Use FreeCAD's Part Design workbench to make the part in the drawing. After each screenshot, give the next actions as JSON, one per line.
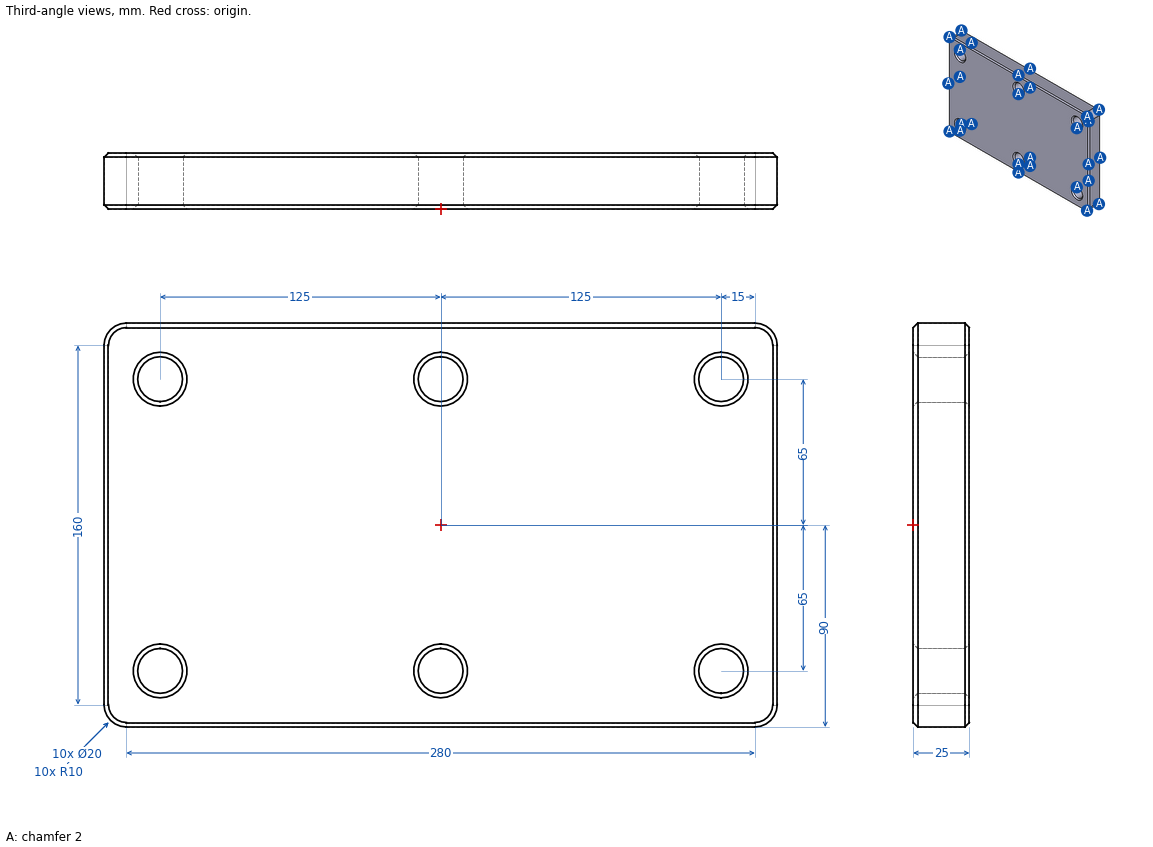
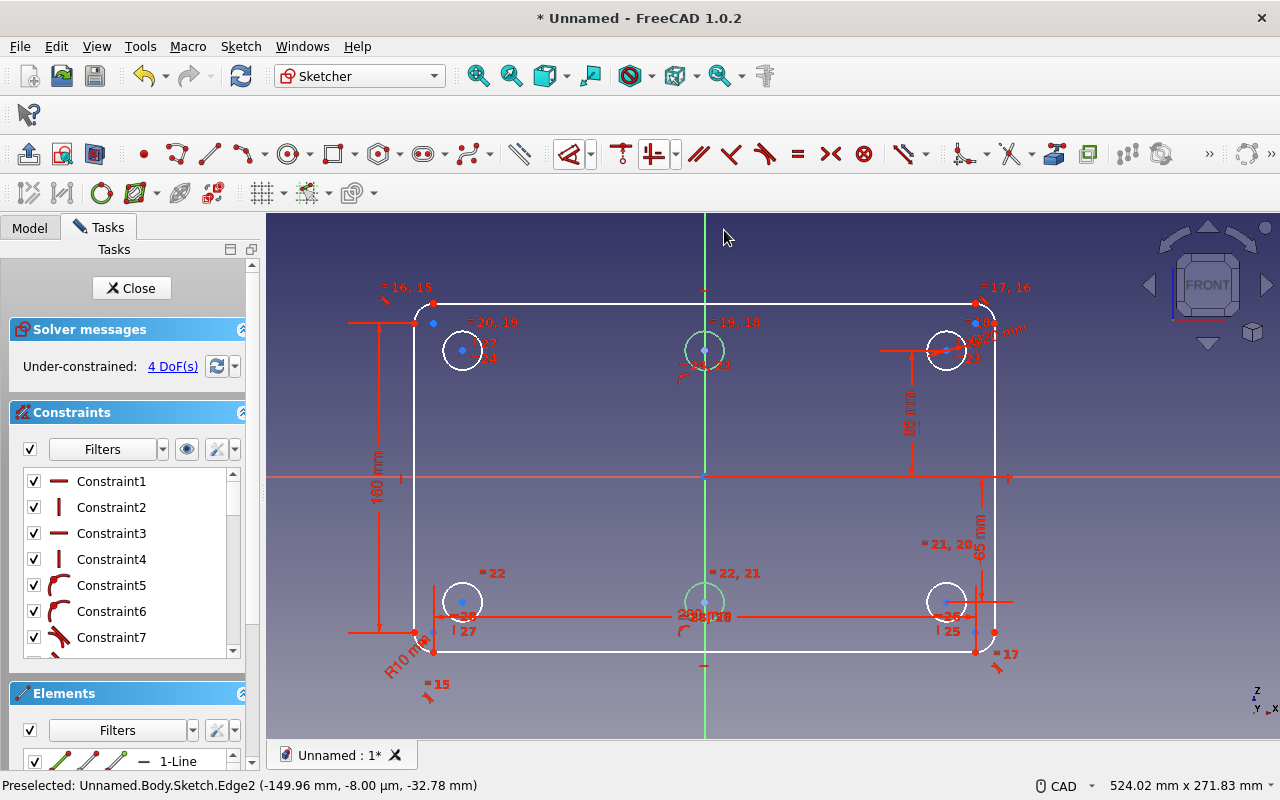
{"action": "left_click", "coordinate": [976, 652]}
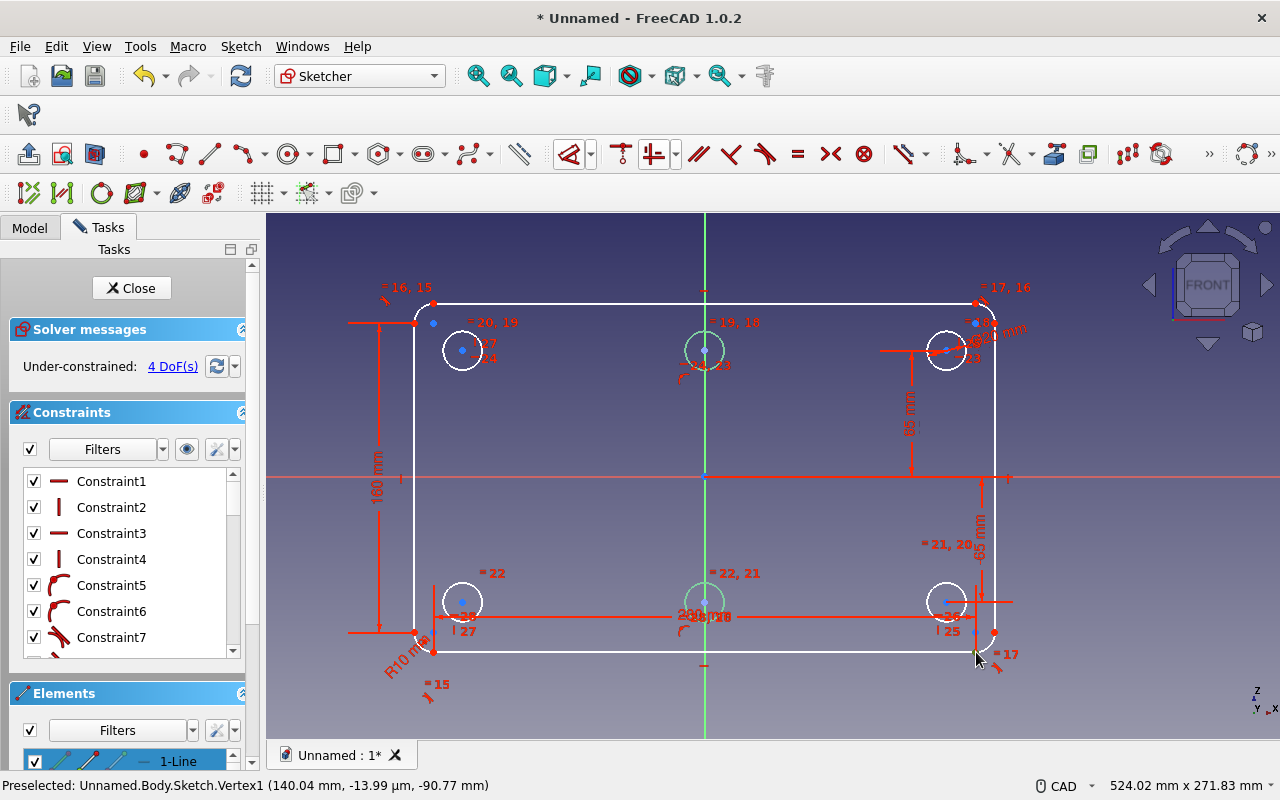
{"action": "left_click", "coordinate": [590, 154]}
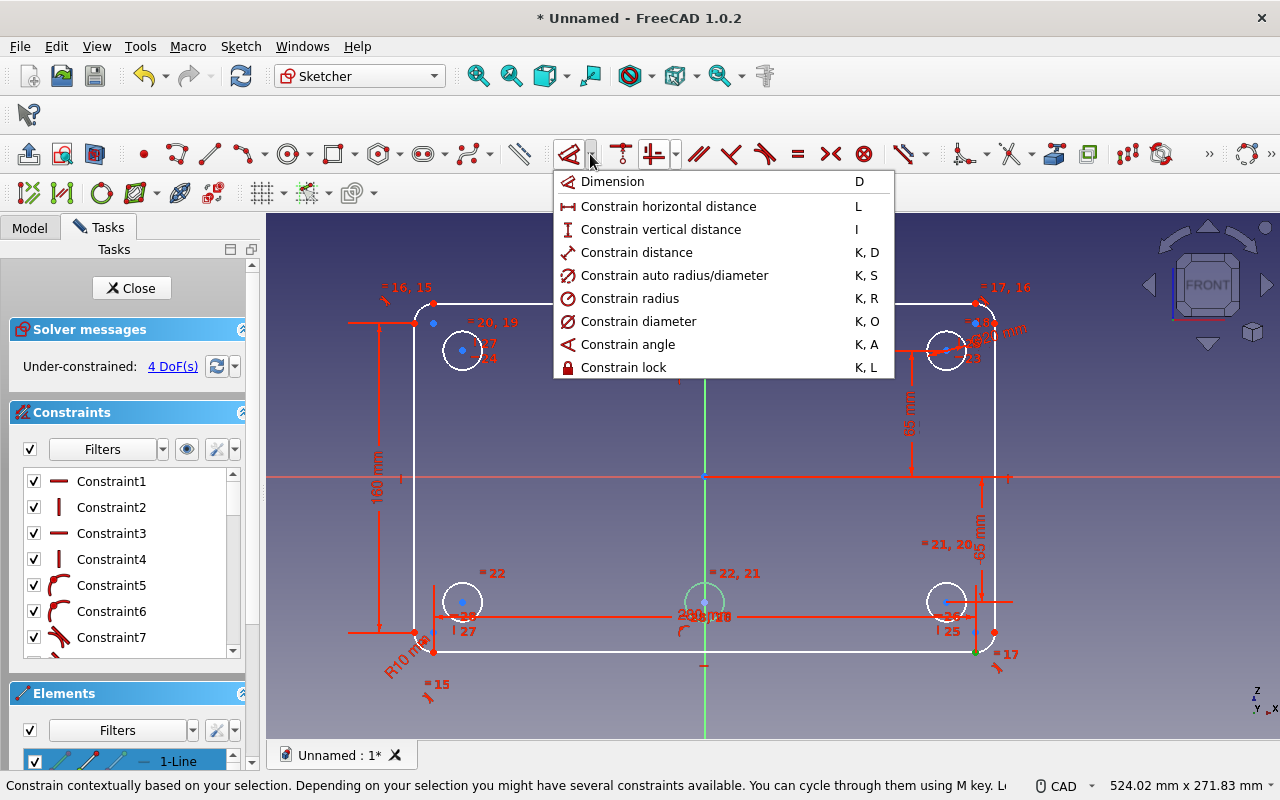
{"action": "left_click", "coordinate": [724, 230]}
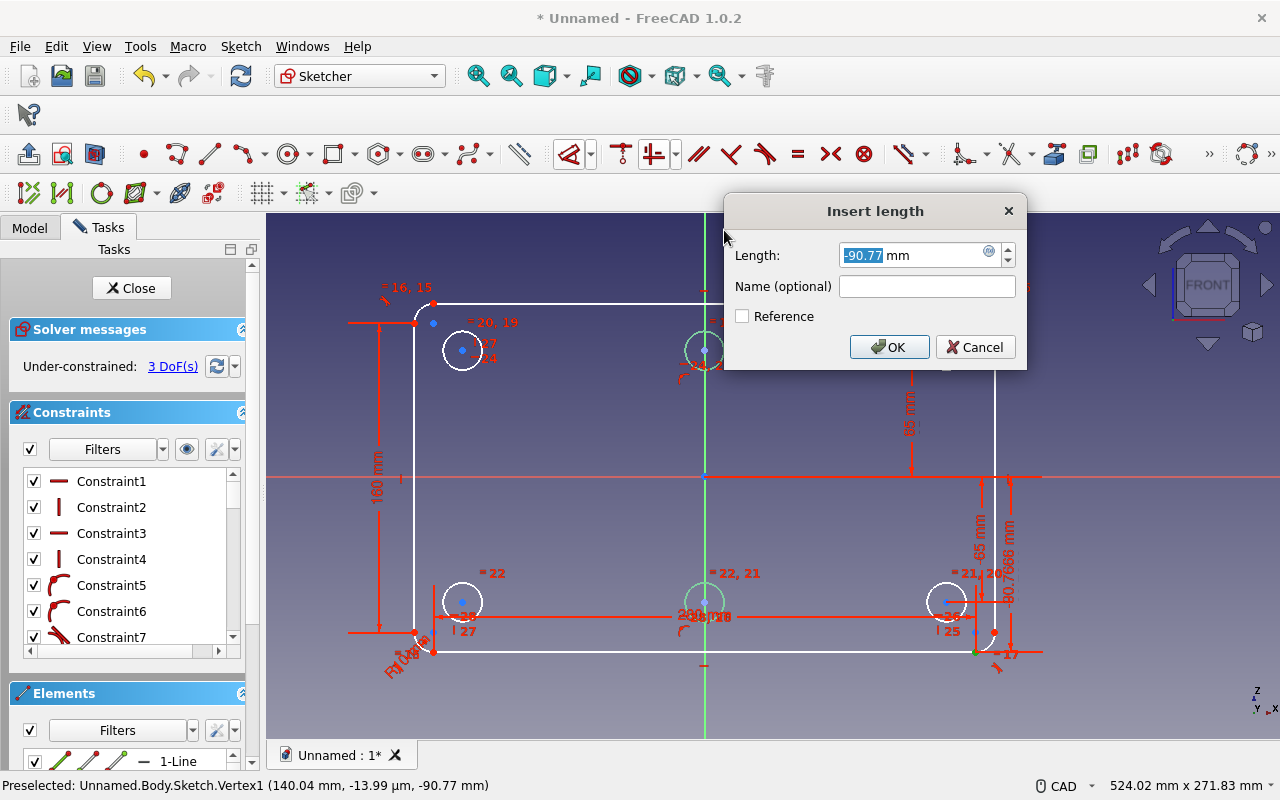
{"action": "type", "text": "-90"}
{"action": "key", "text": "Return"}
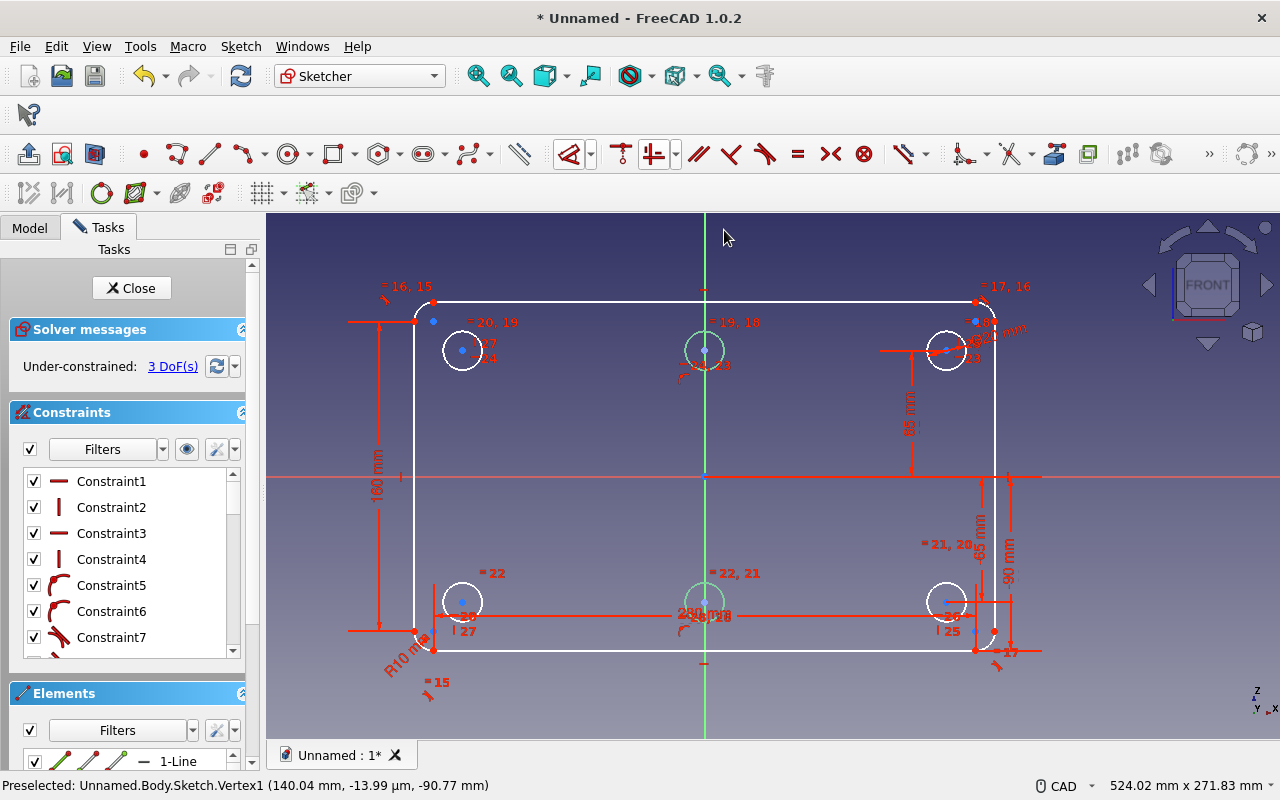
{"action": "left_click", "coordinate": [947, 351]}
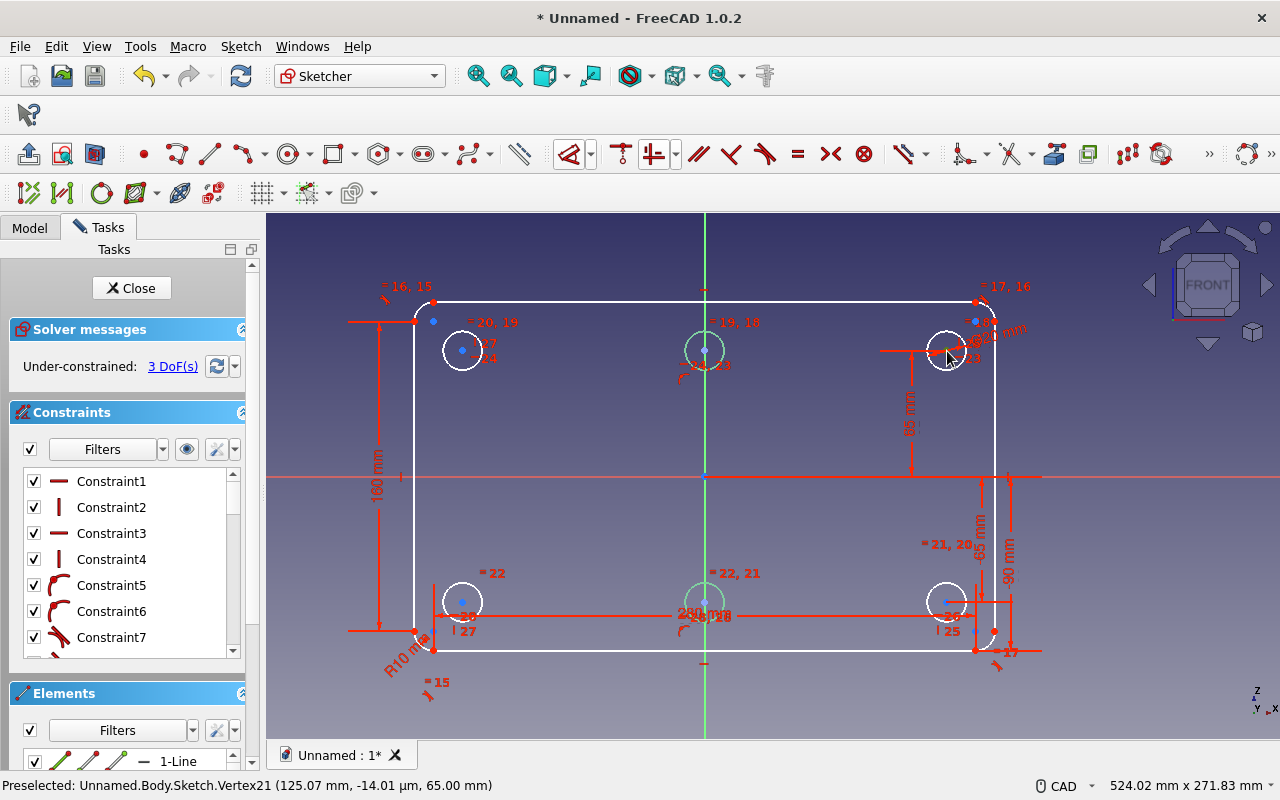
{"action": "key", "text": "l"}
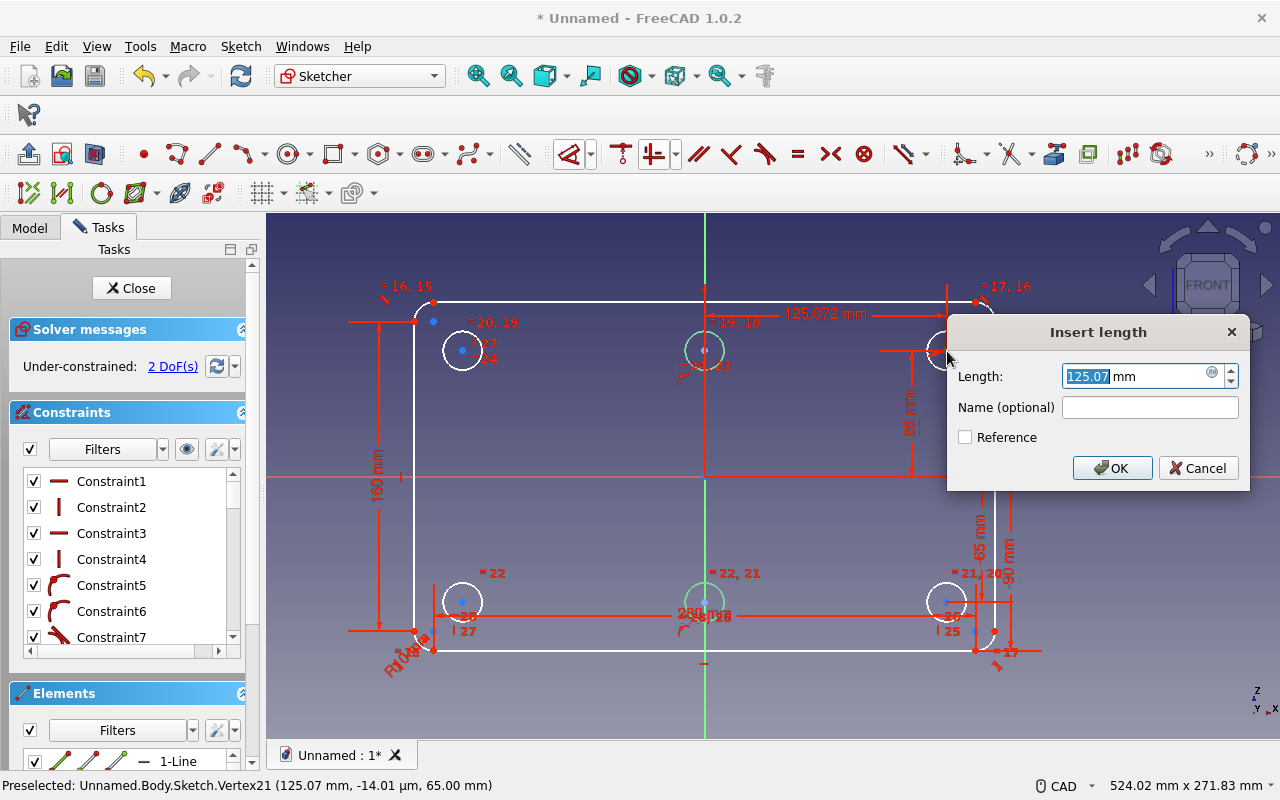
{"action": "type", "text": "125"}
{"action": "key", "text": "Return"}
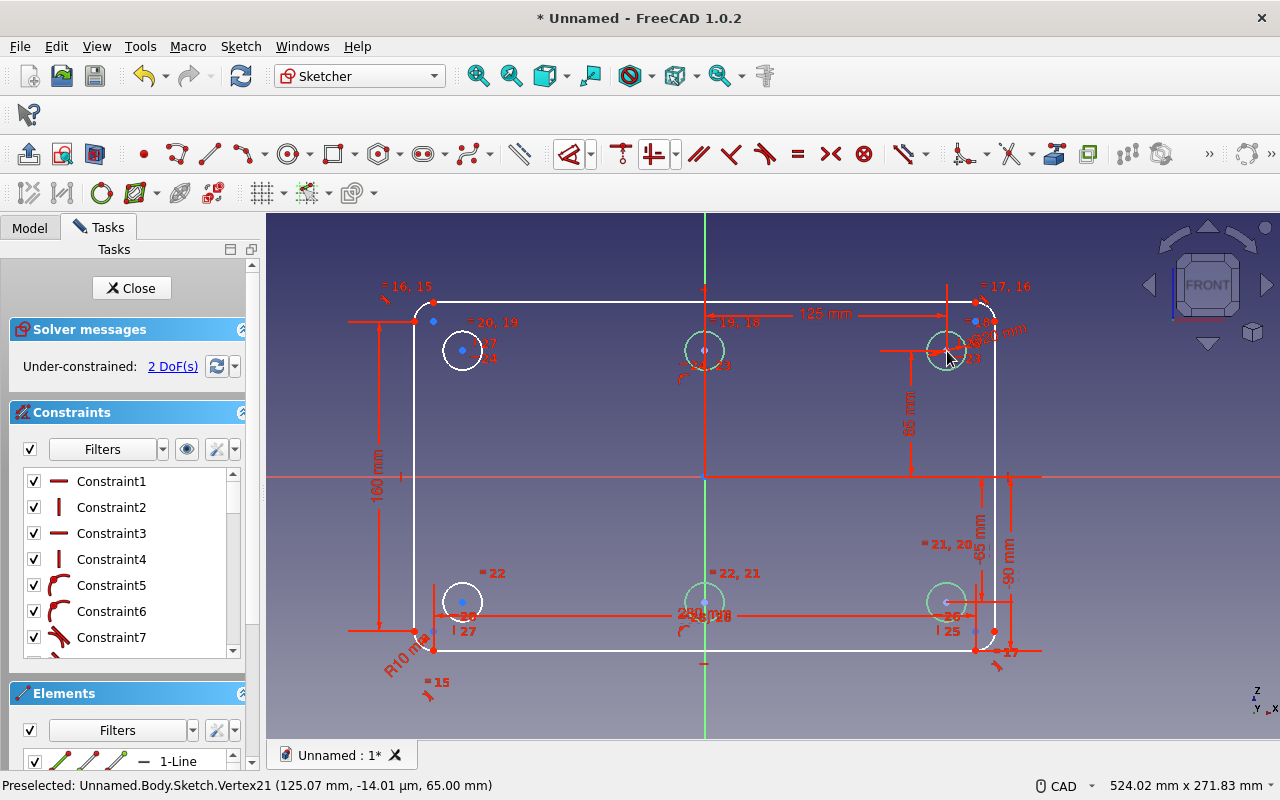
{"action": "left_click", "coordinate": [463, 351]}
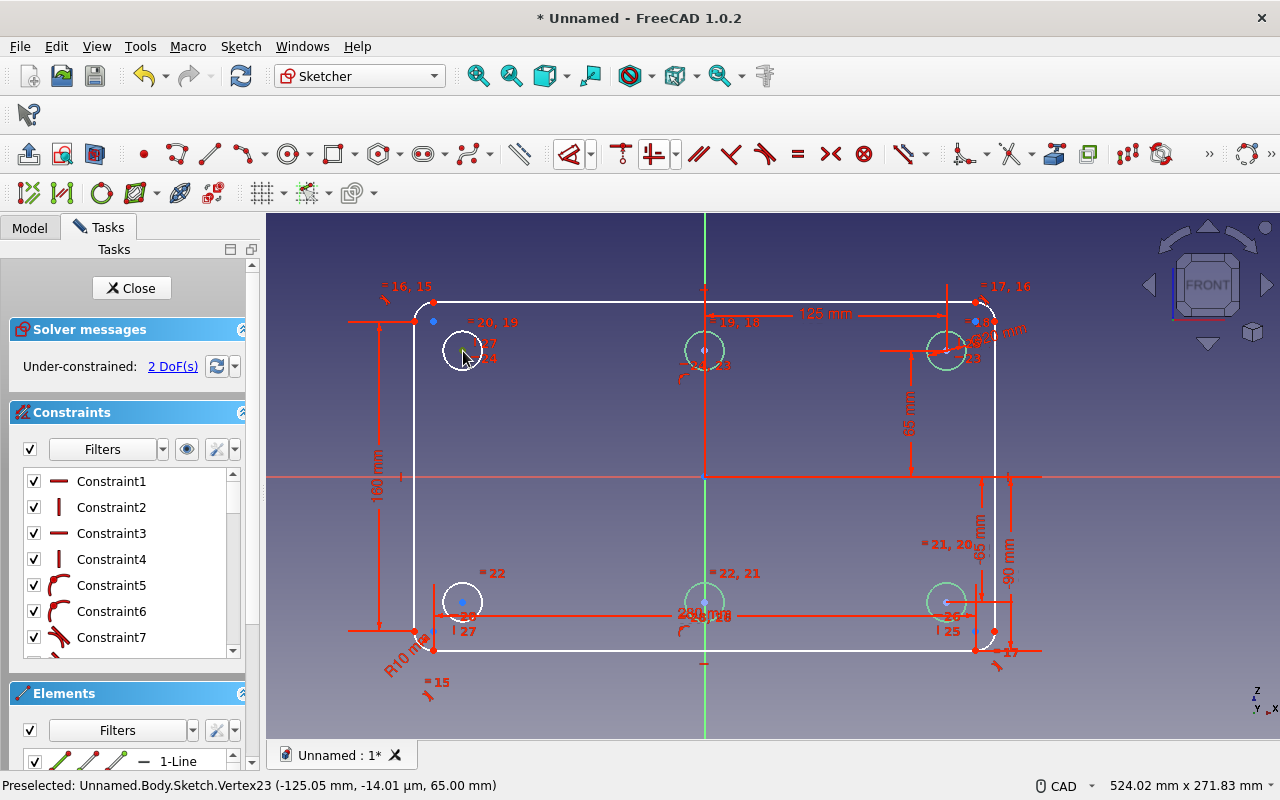
{"action": "left_click", "coordinate": [590, 154]}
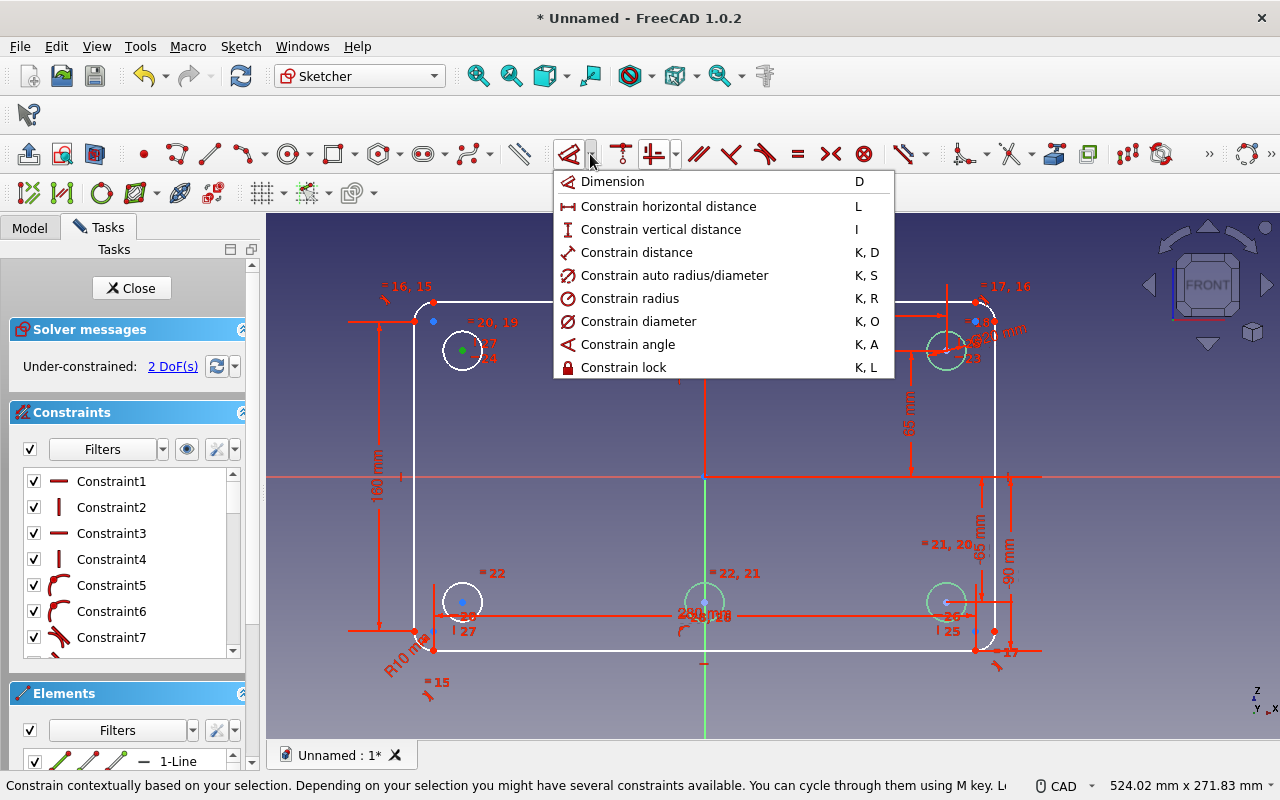
{"action": "left_click", "coordinate": [724, 206]}